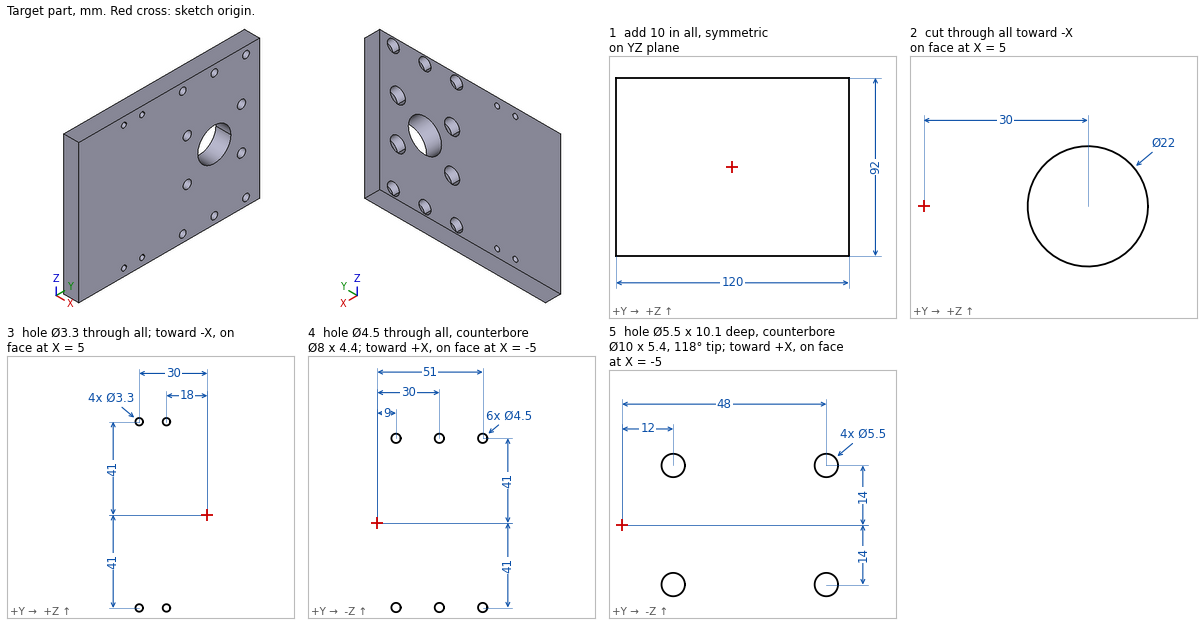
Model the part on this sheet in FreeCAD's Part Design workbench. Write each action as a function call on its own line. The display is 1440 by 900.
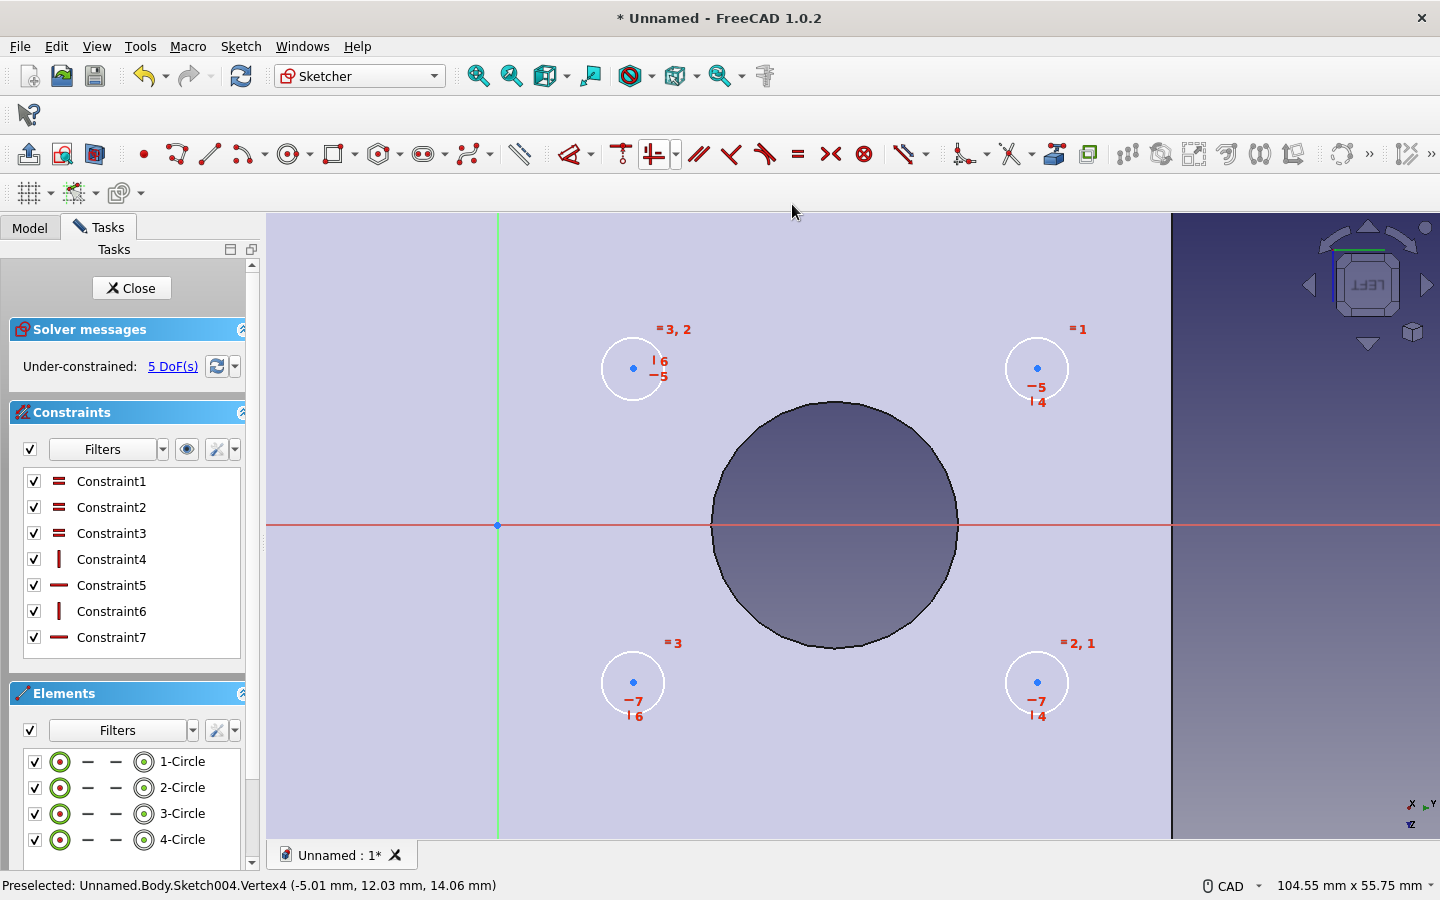
click(1059, 347)
click(1082, 324)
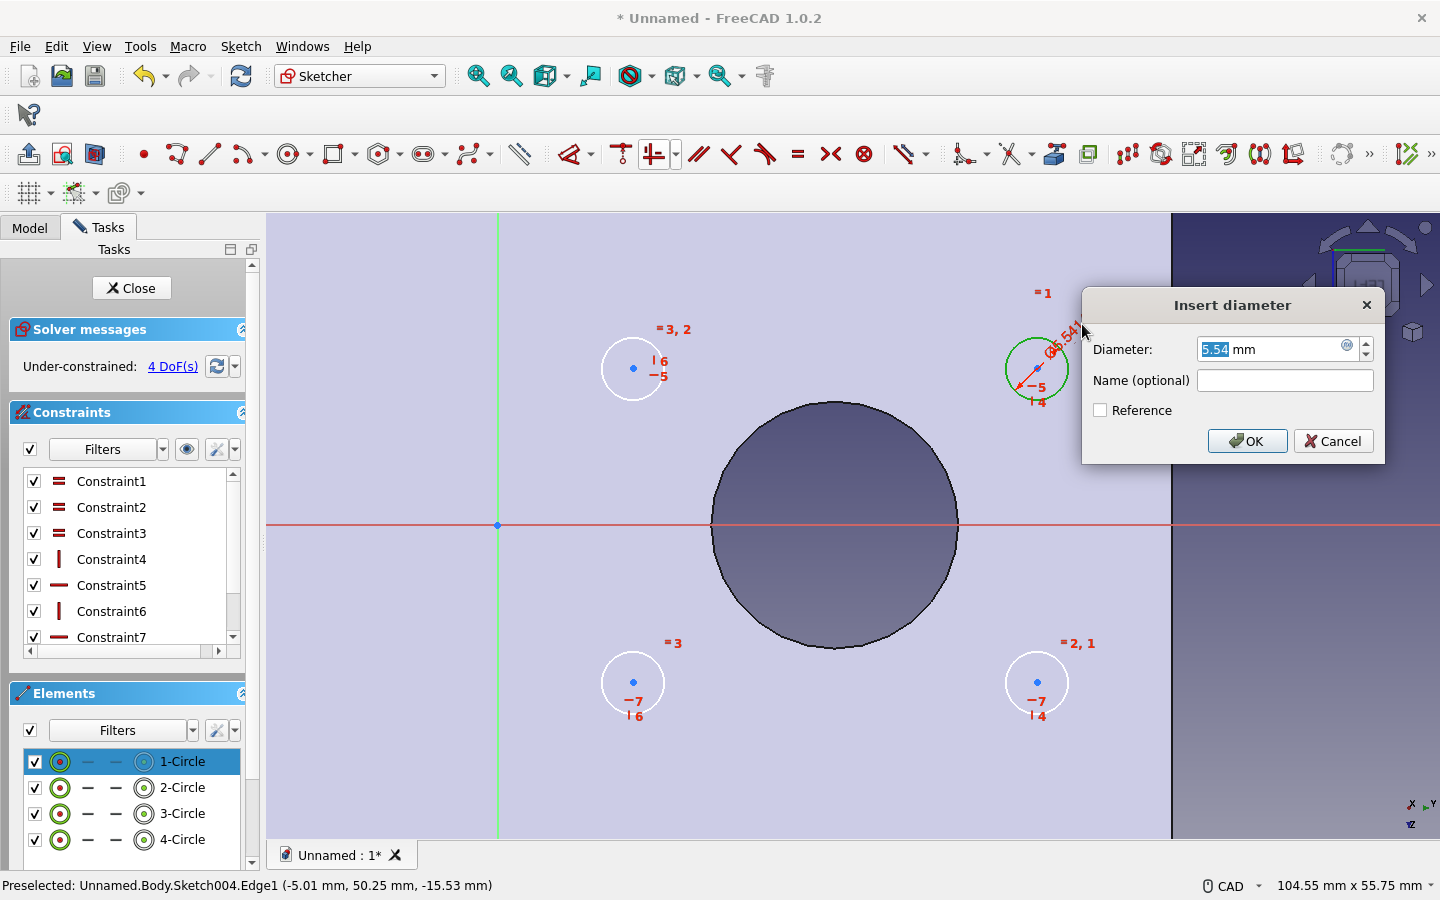
text(5.5)
key(Return)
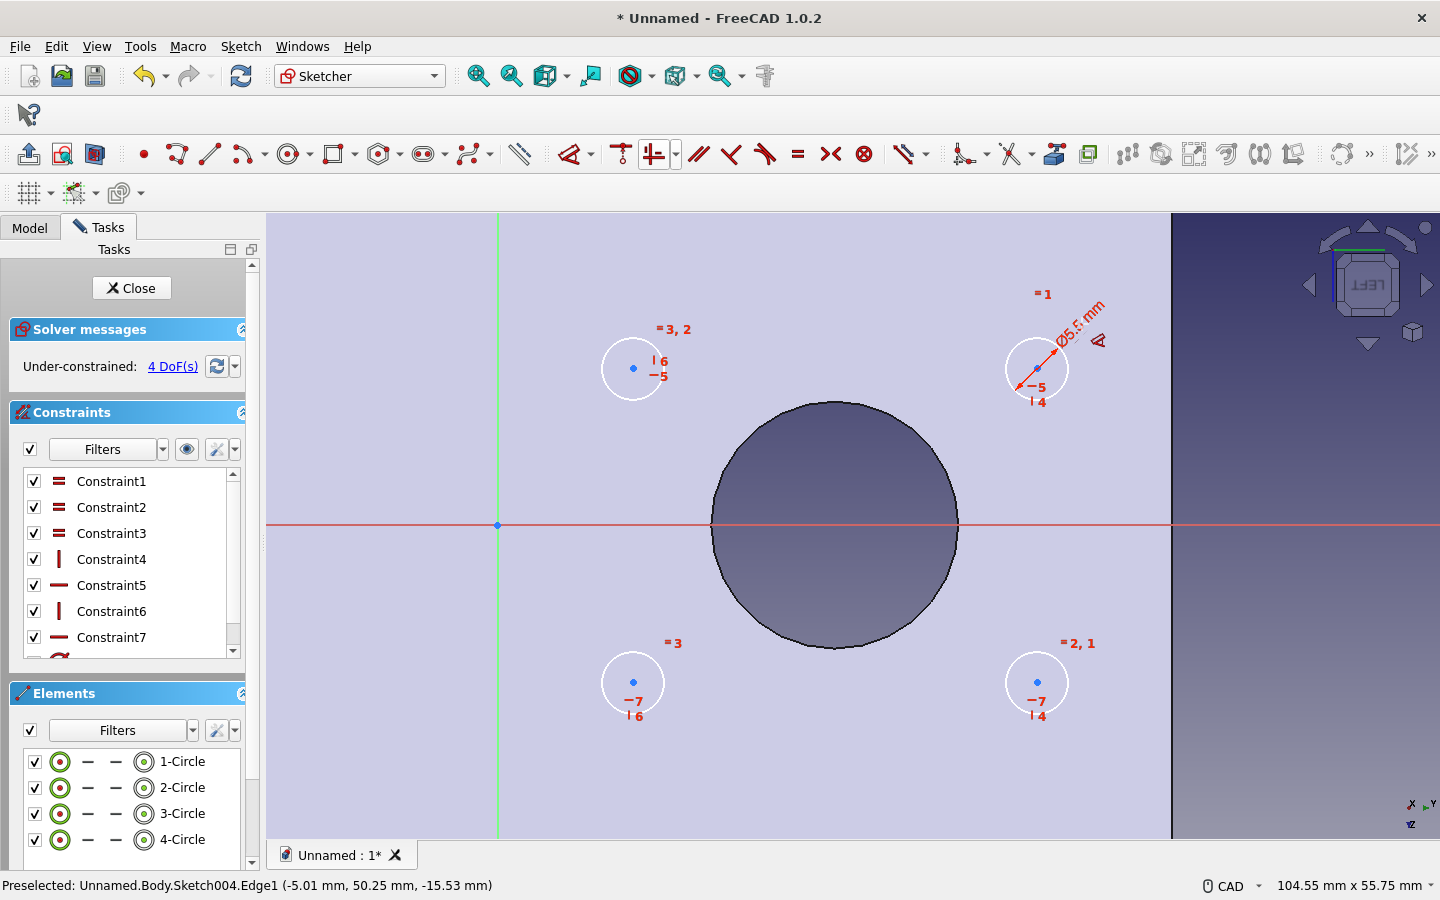
click(1037, 369)
click(767, 335)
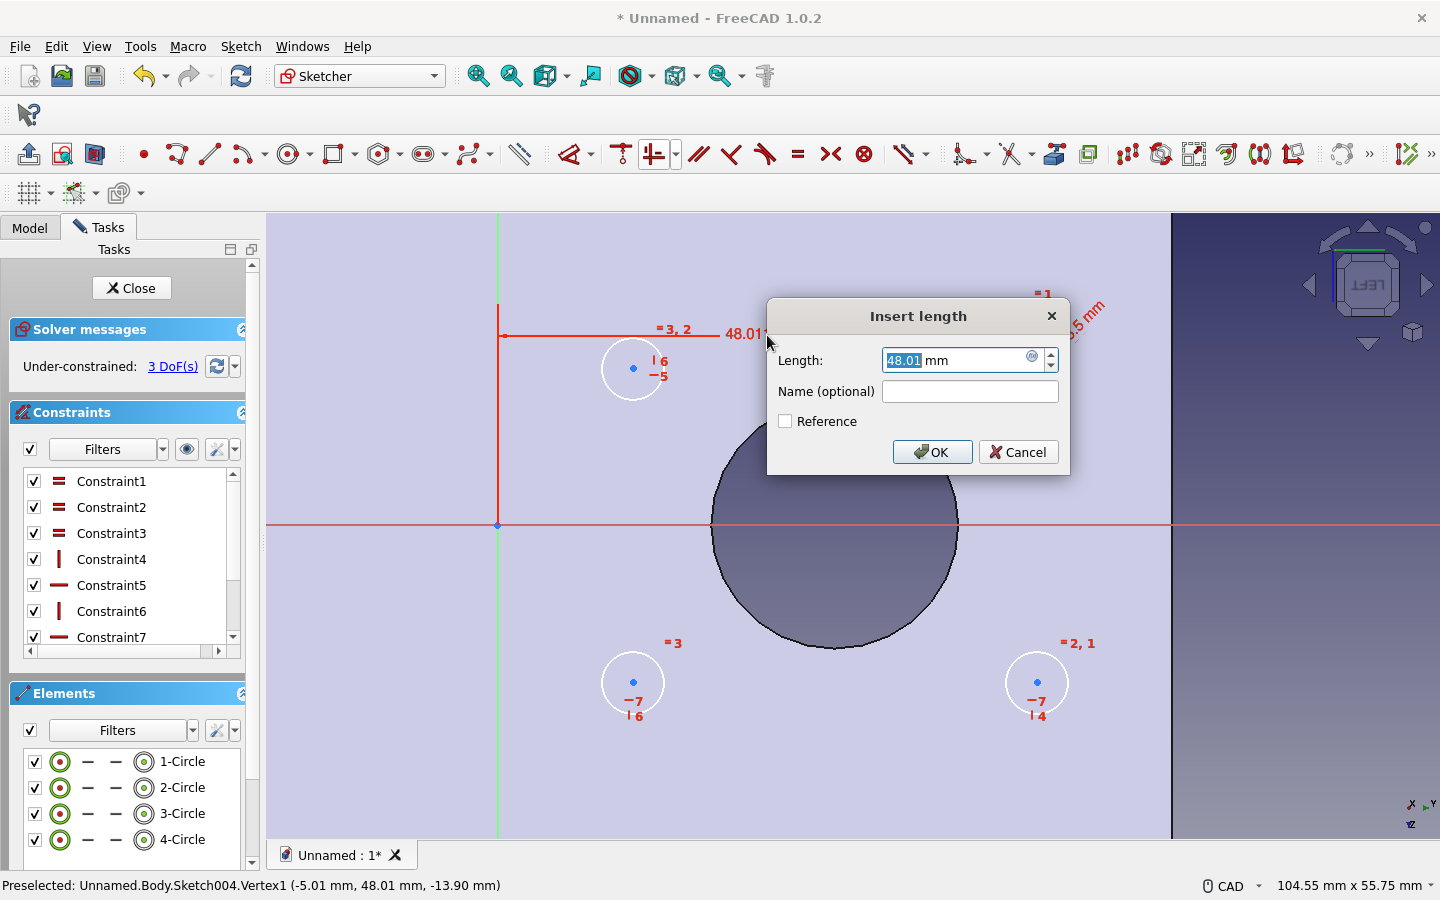
text(48)
key(Return)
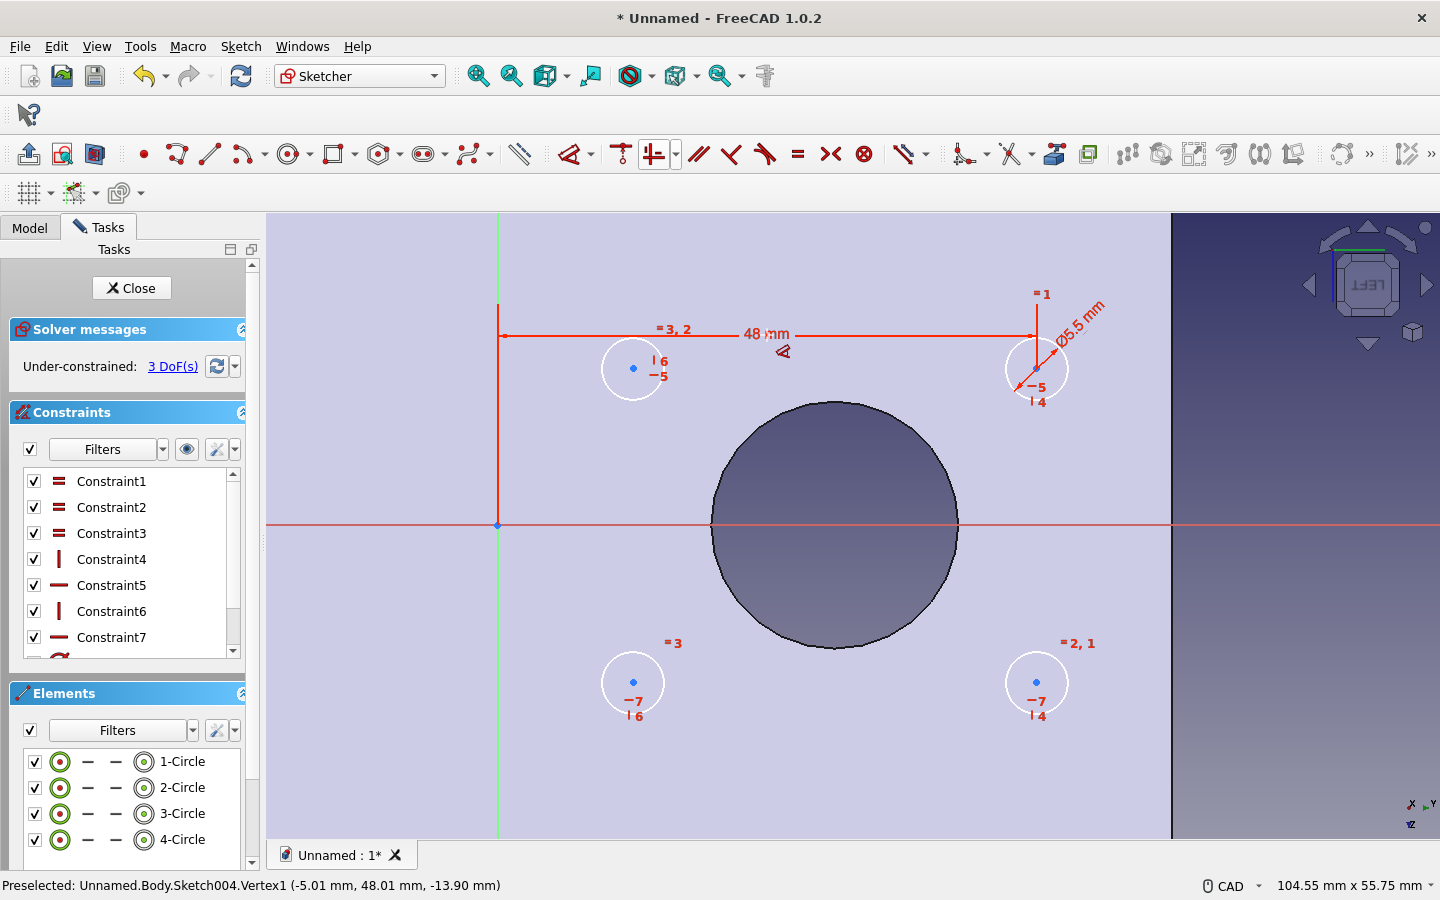
click(1037, 369)
click(464, 447)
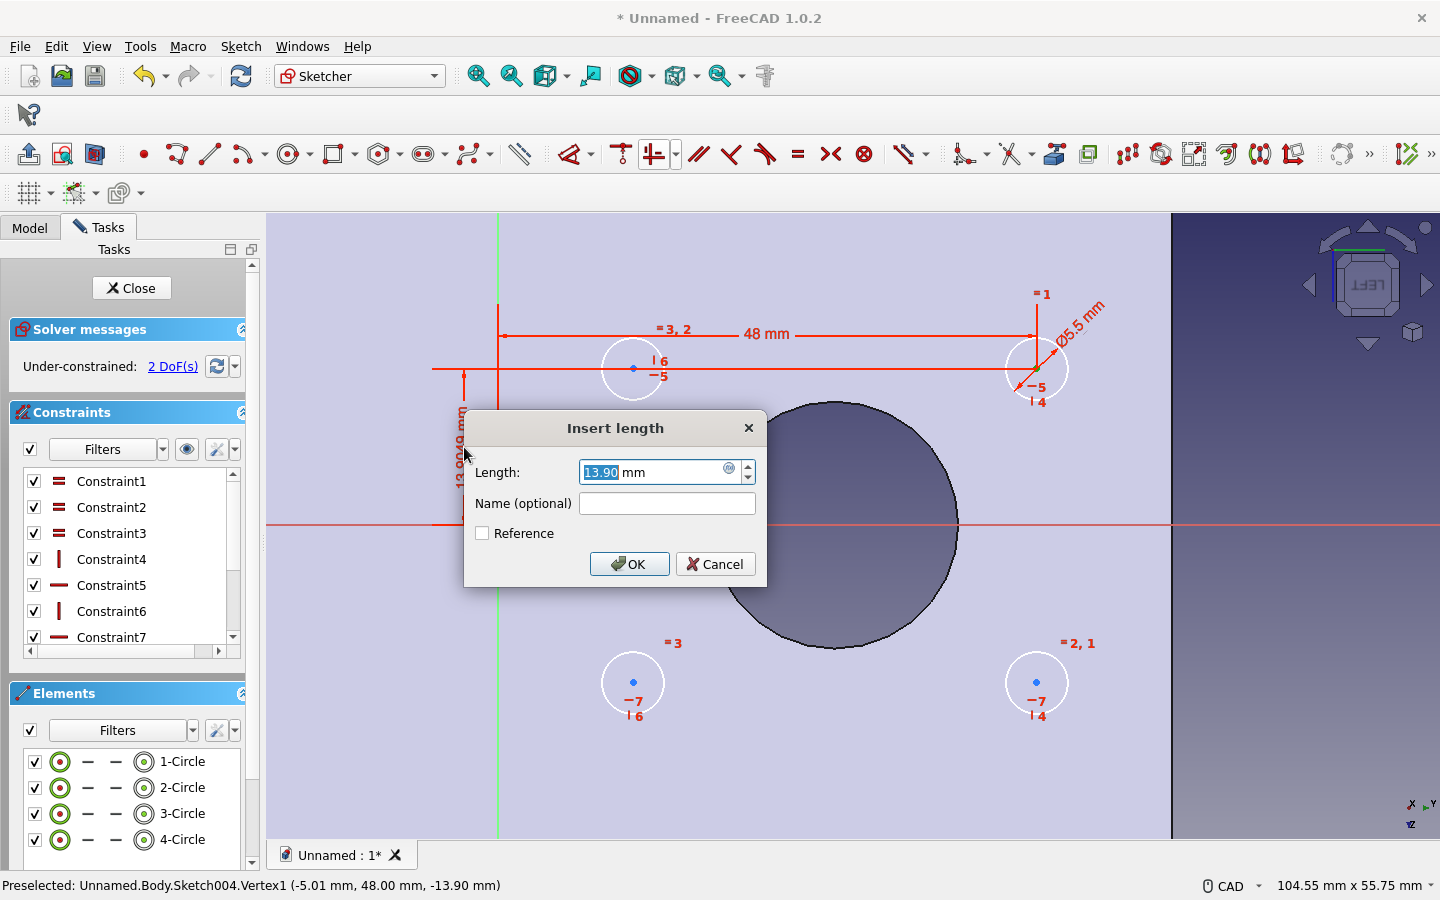
text(14)
key(Return)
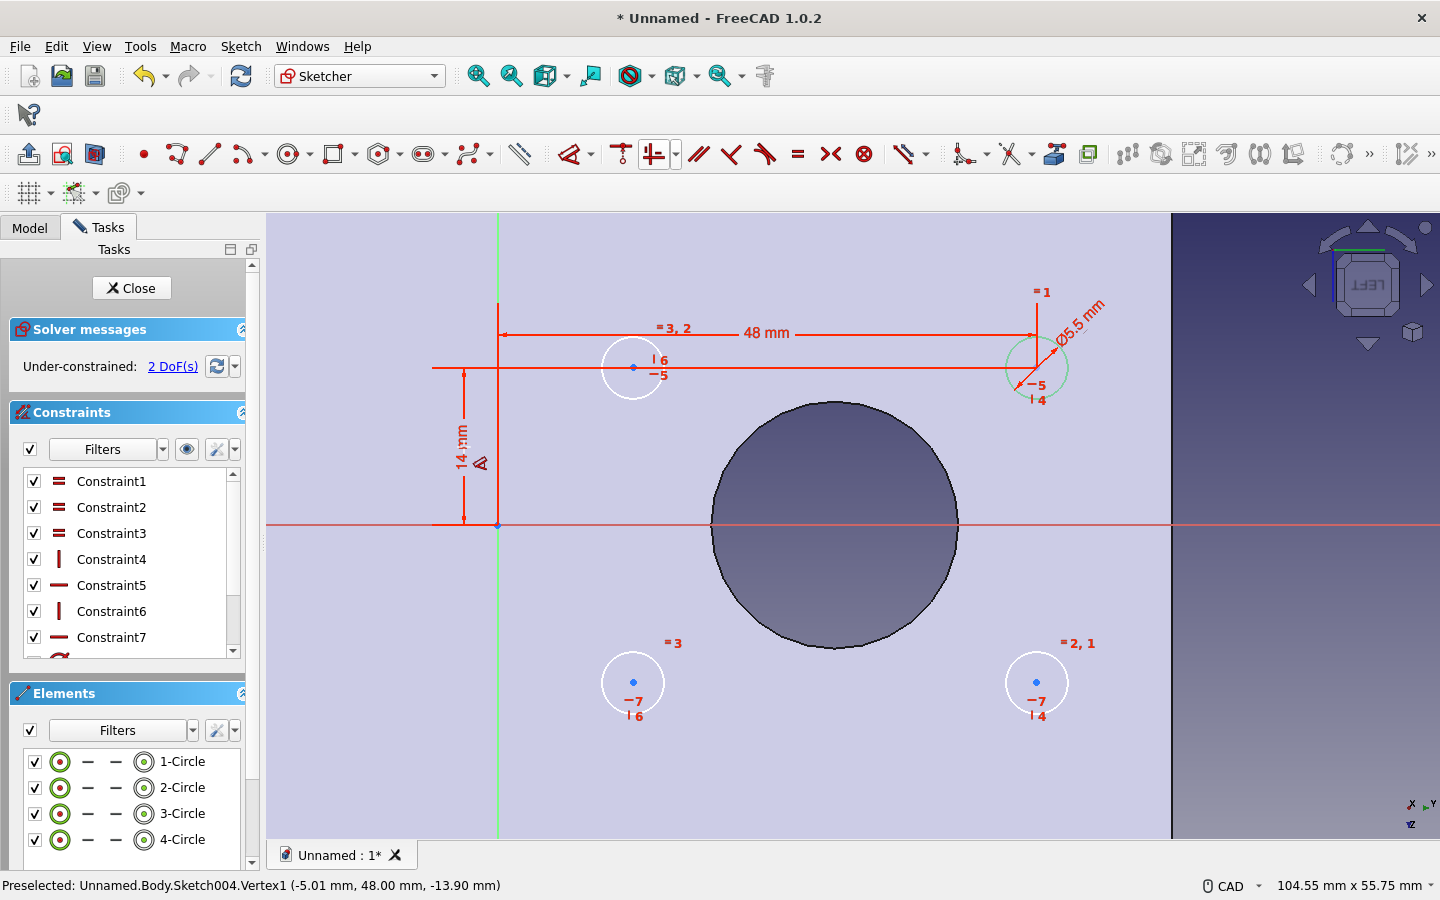
click(1037, 683)
click(464, 604)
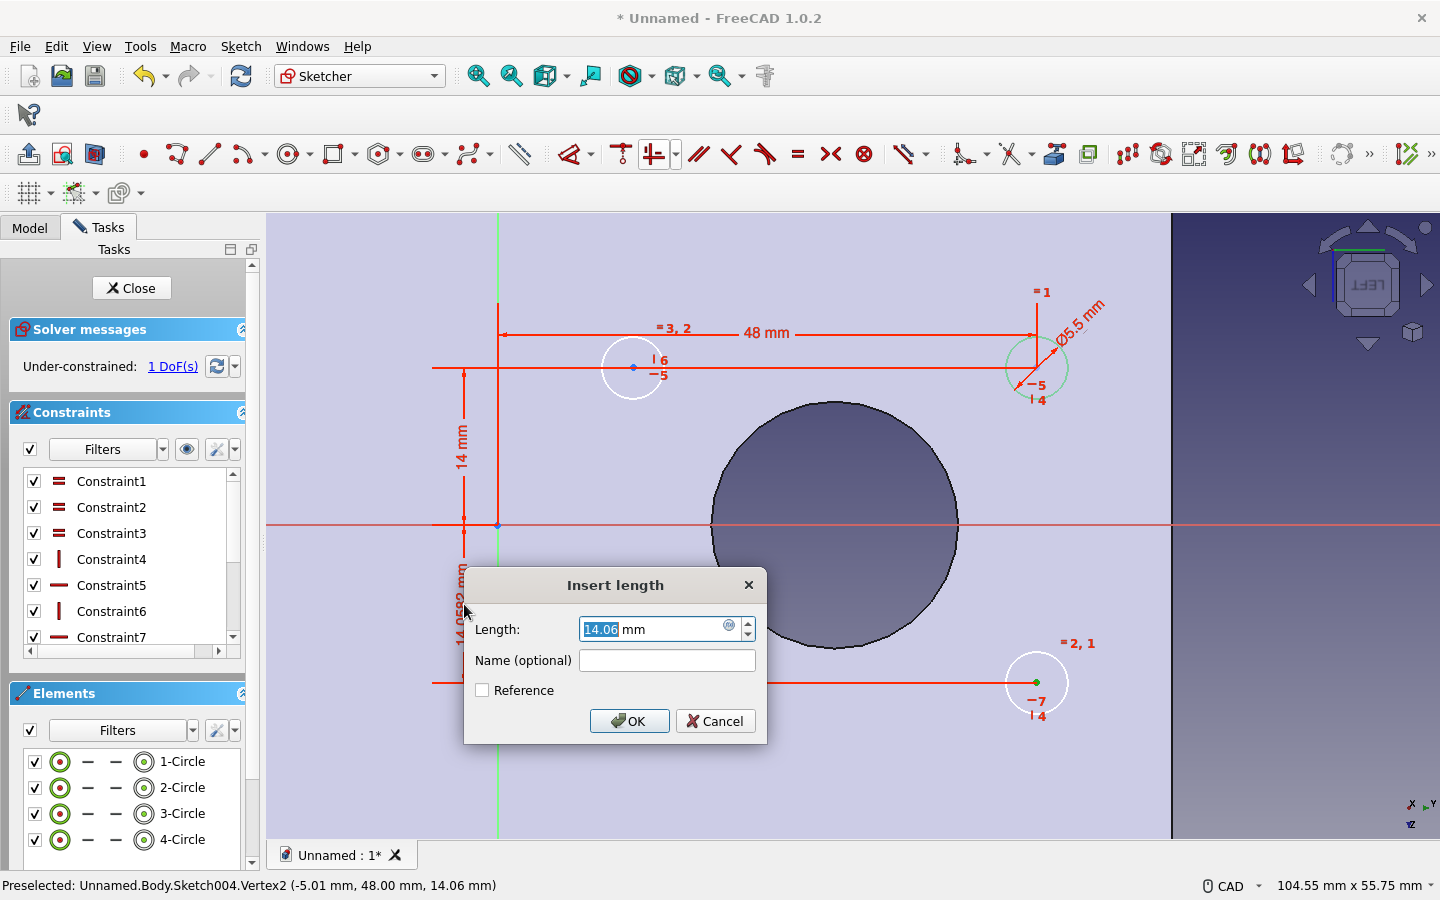
text(14)
key(Return)